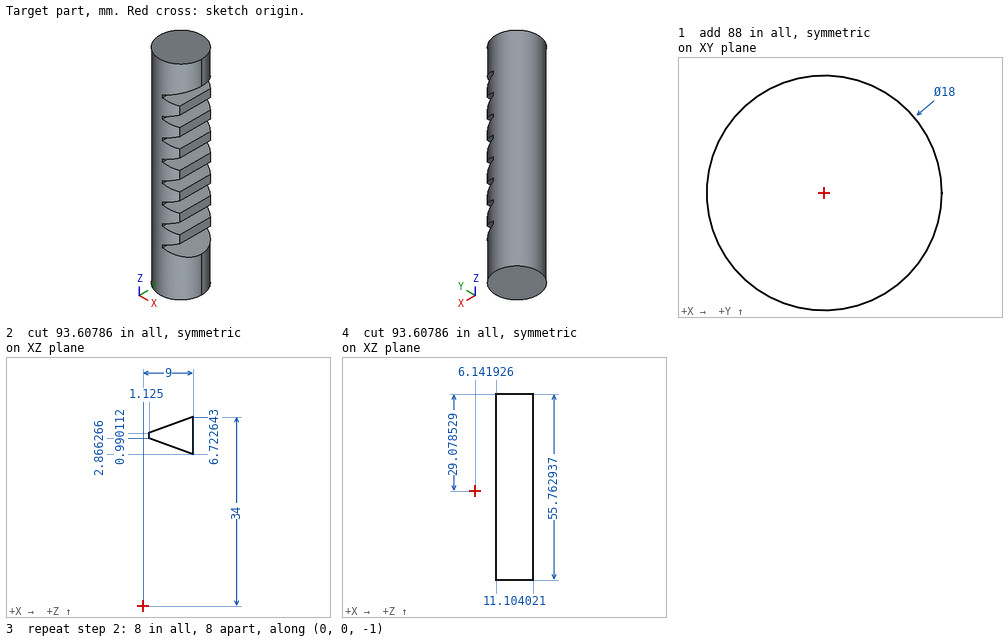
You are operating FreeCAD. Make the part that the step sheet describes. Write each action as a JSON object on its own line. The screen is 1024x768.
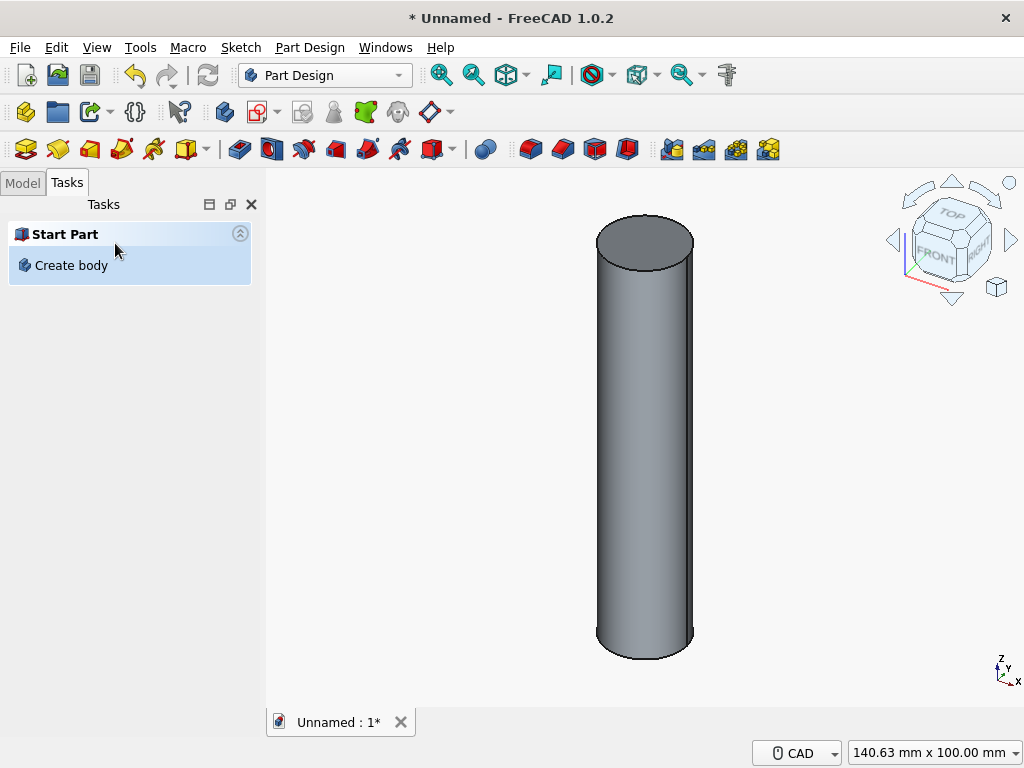
{"action": "left_click", "coordinate": [258, 112]}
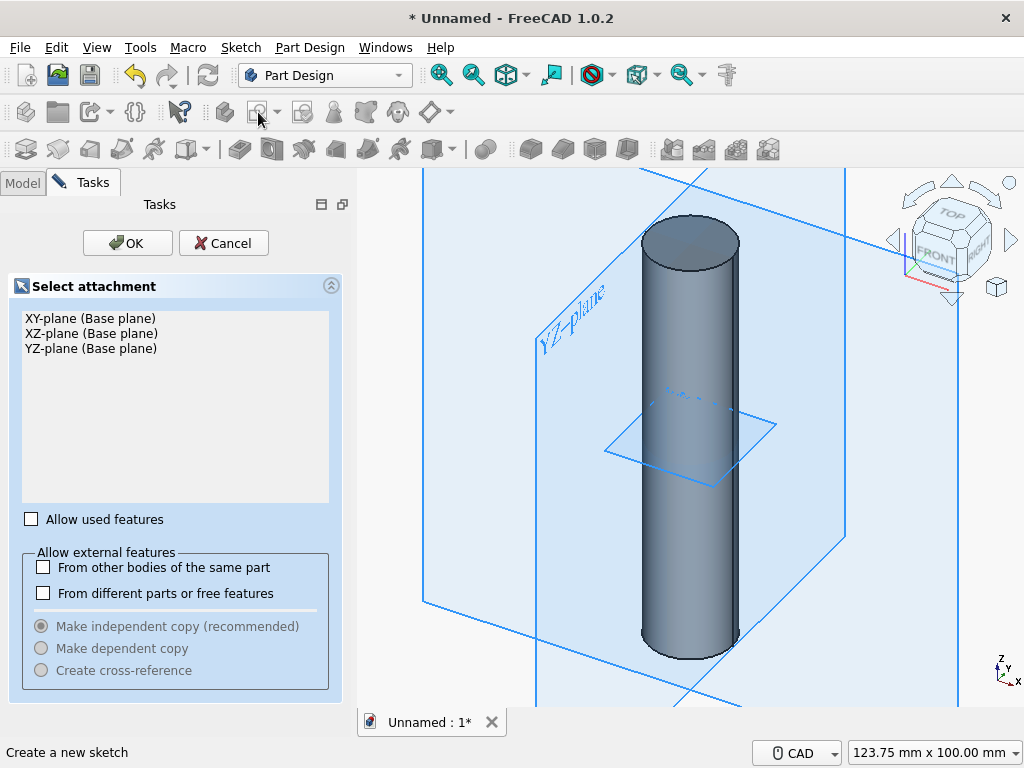
{"action": "left_click", "coordinate": [82, 334]}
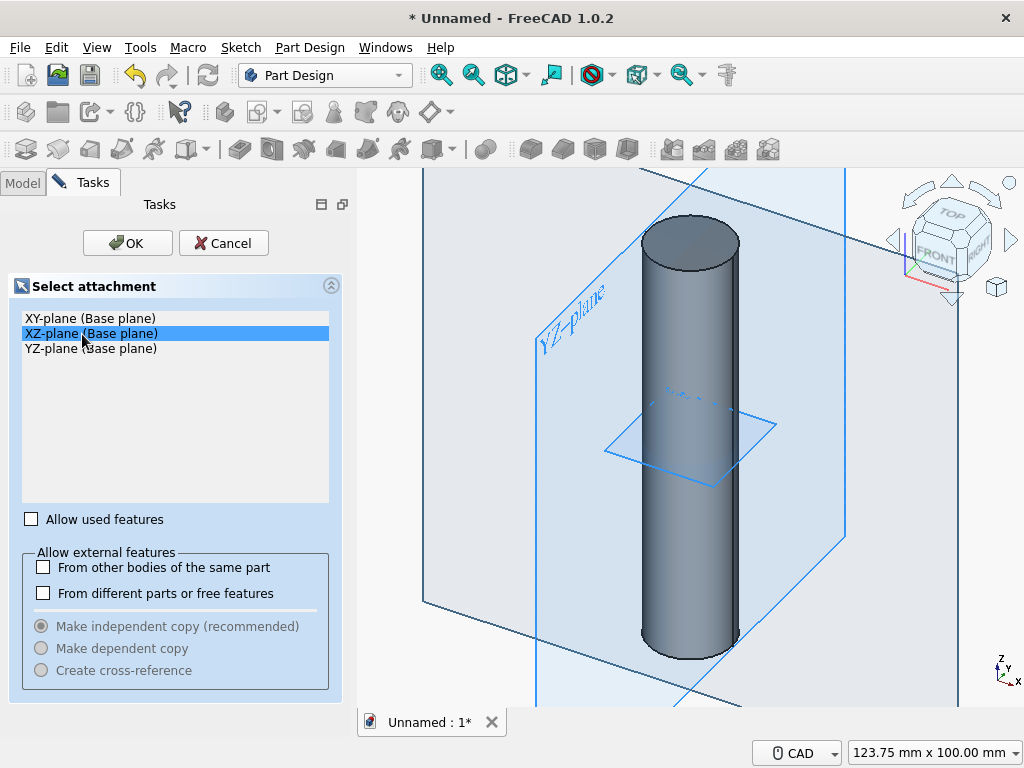
{"action": "left_click", "coordinate": [128, 243]}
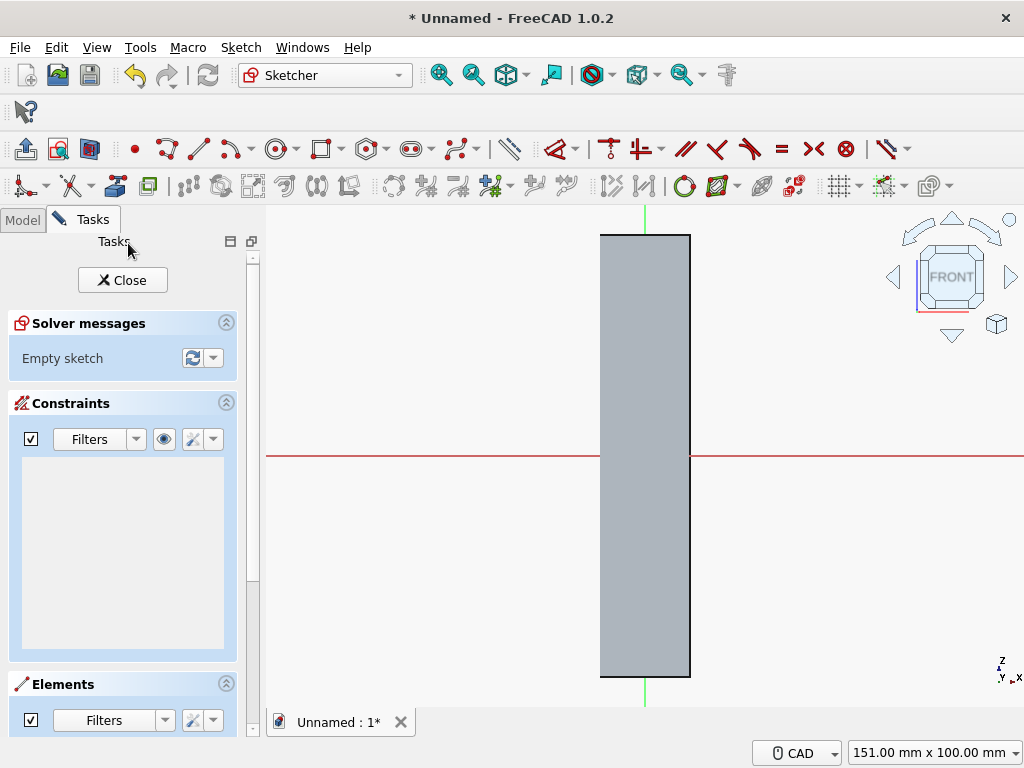
{"action": "left_click", "coordinate": [90, 150]}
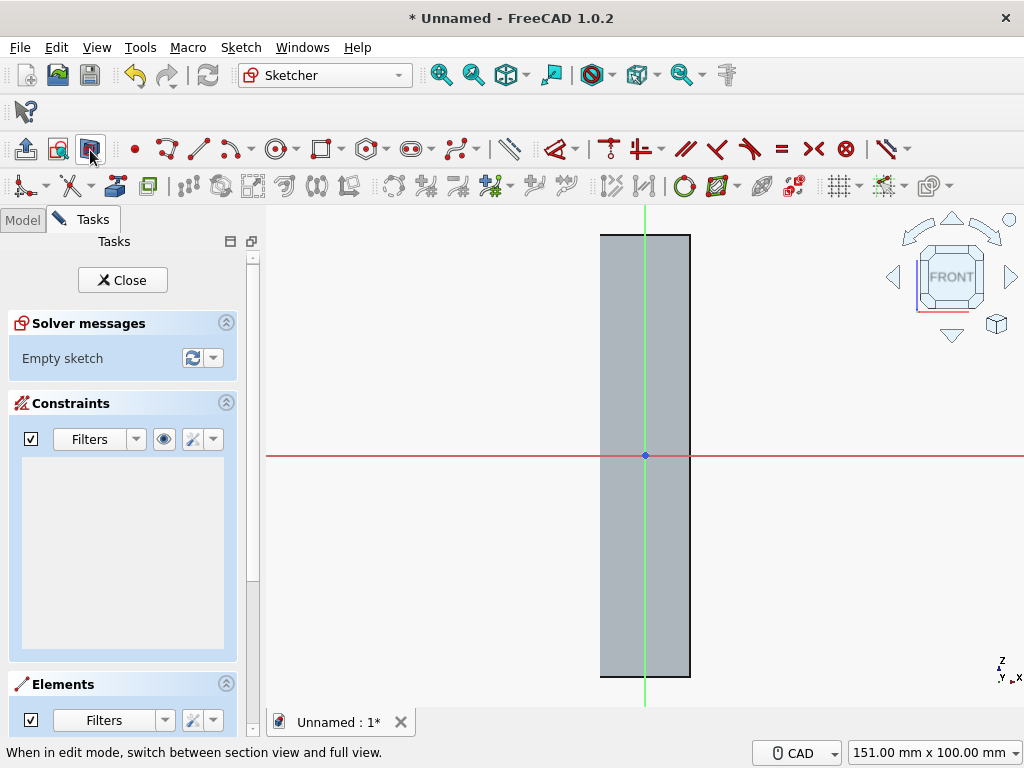
{"action": "scroll", "coordinate": [682, 283], "scroll_direction": "up", "scroll_amount": 11}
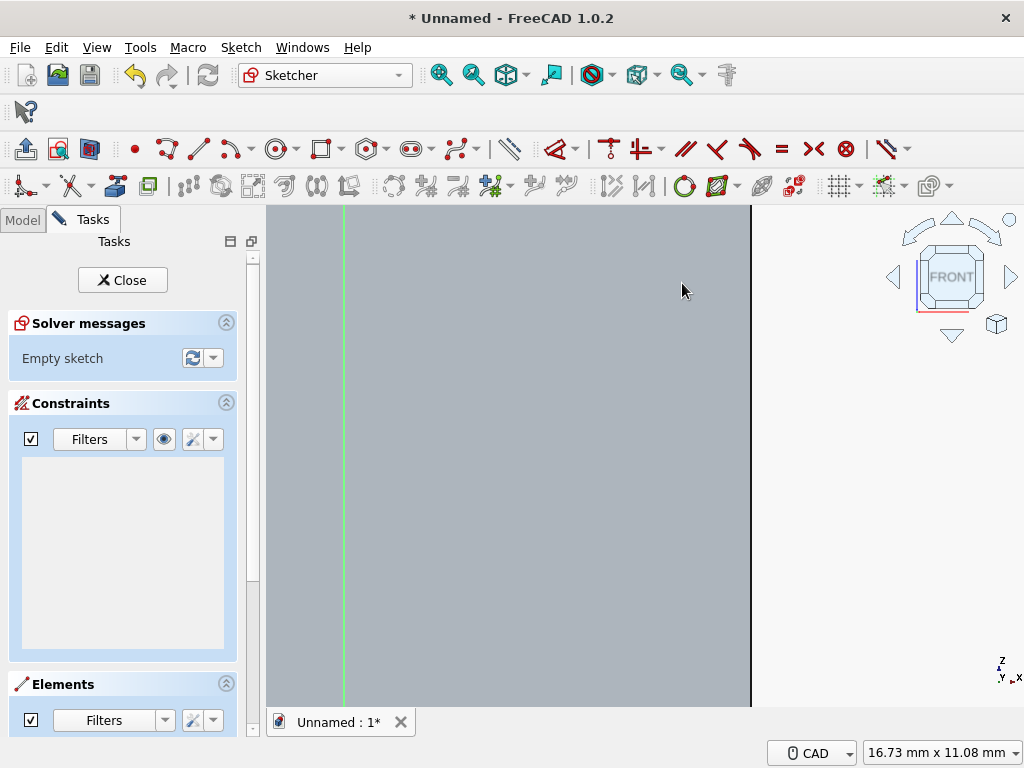
{"action": "key", "text": "g m"}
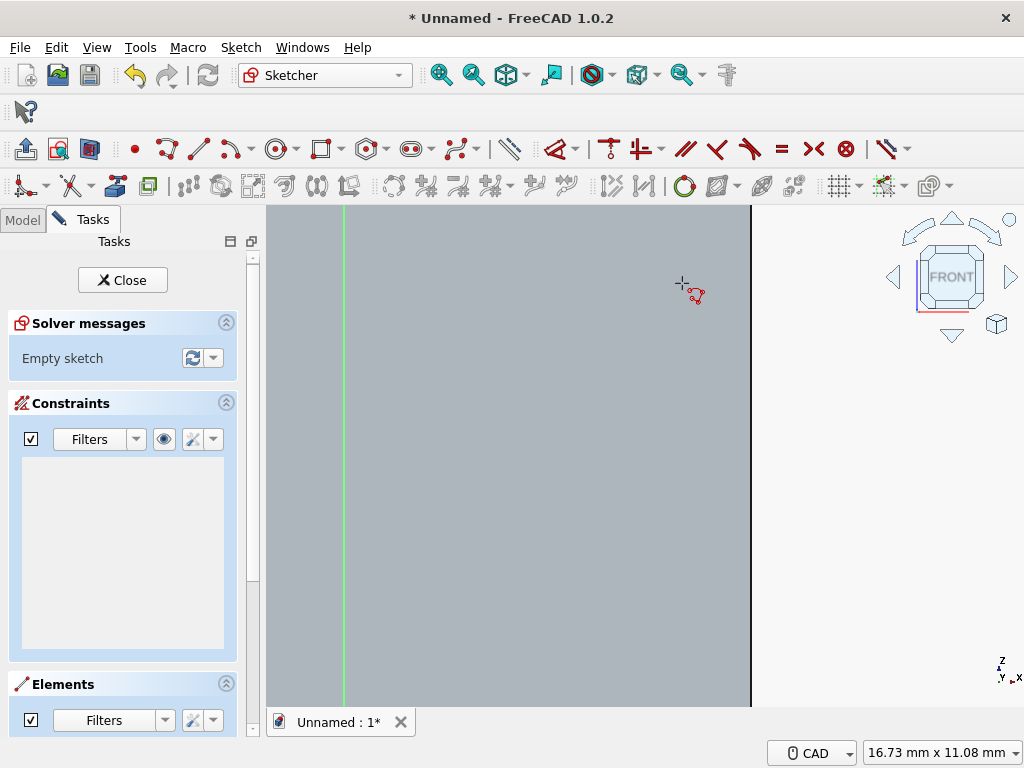
{"action": "left_click", "coordinate": [751, 607]}
{"action": "left_click", "coordinate": [395, 477]}
{"action": "left_click", "coordinate": [395, 433]}
{"action": "left_click", "coordinate": [751, 303]}
{"action": "left_click", "coordinate": [751, 608]}
{"action": "key", "text": "Escape"}
{"action": "key", "text": "Escape"}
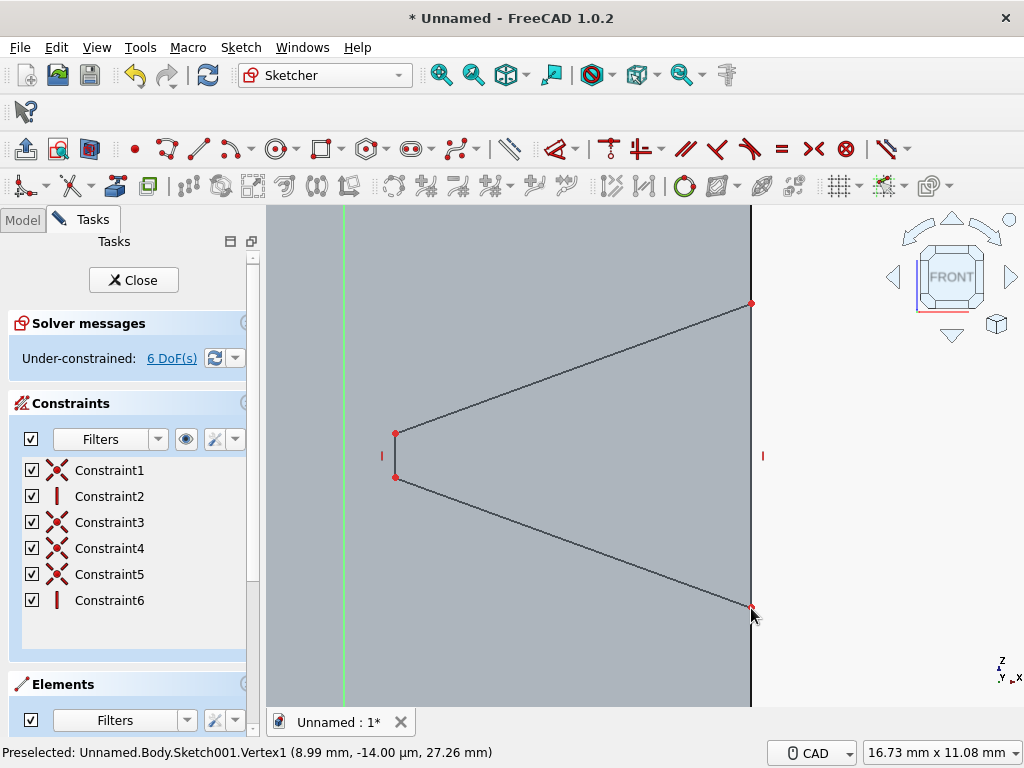
{"action": "left_click", "coordinate": [751, 608]}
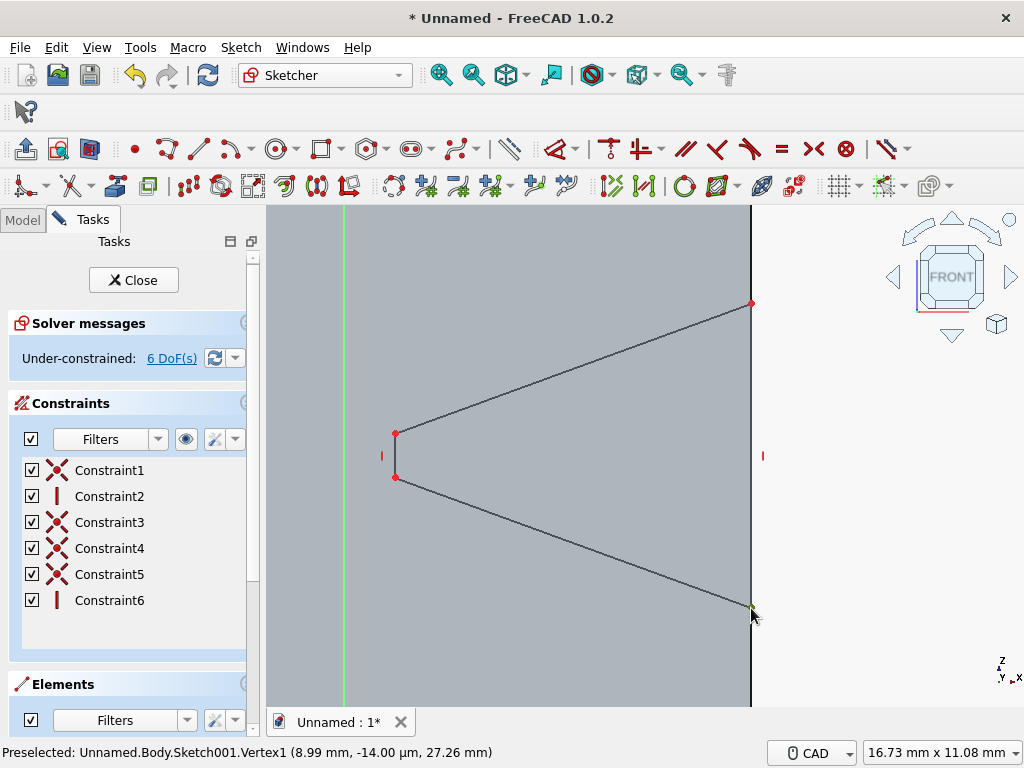
{"action": "left_click", "coordinate": [578, 150]}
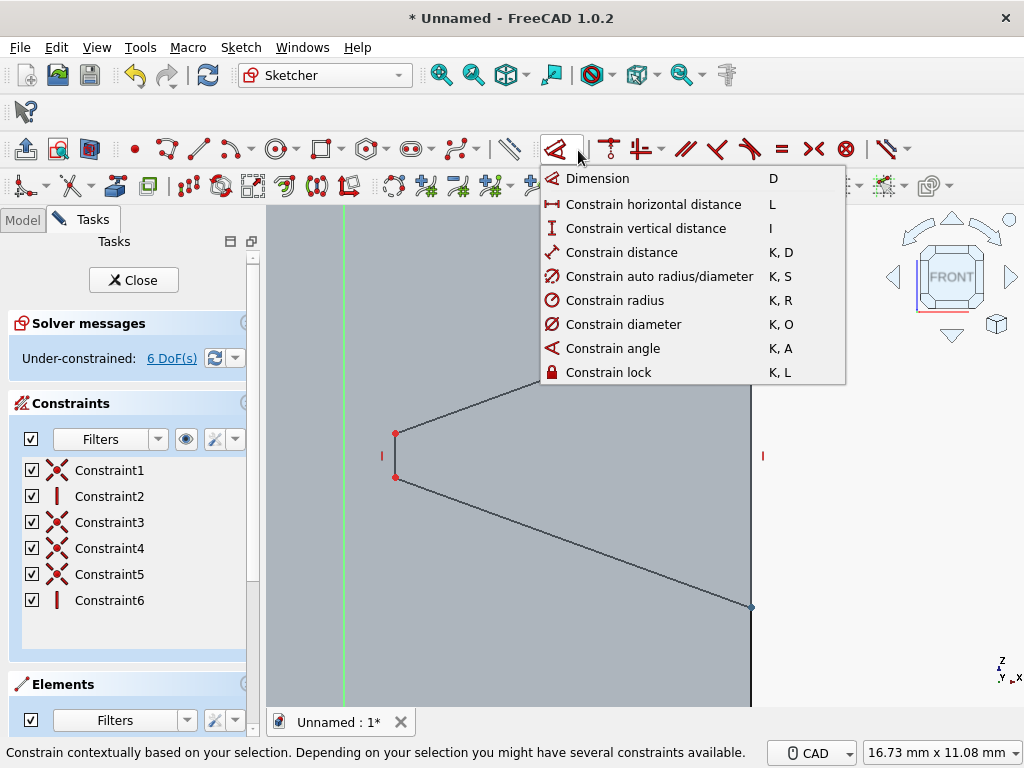
{"action": "left_click", "coordinate": [693, 204]}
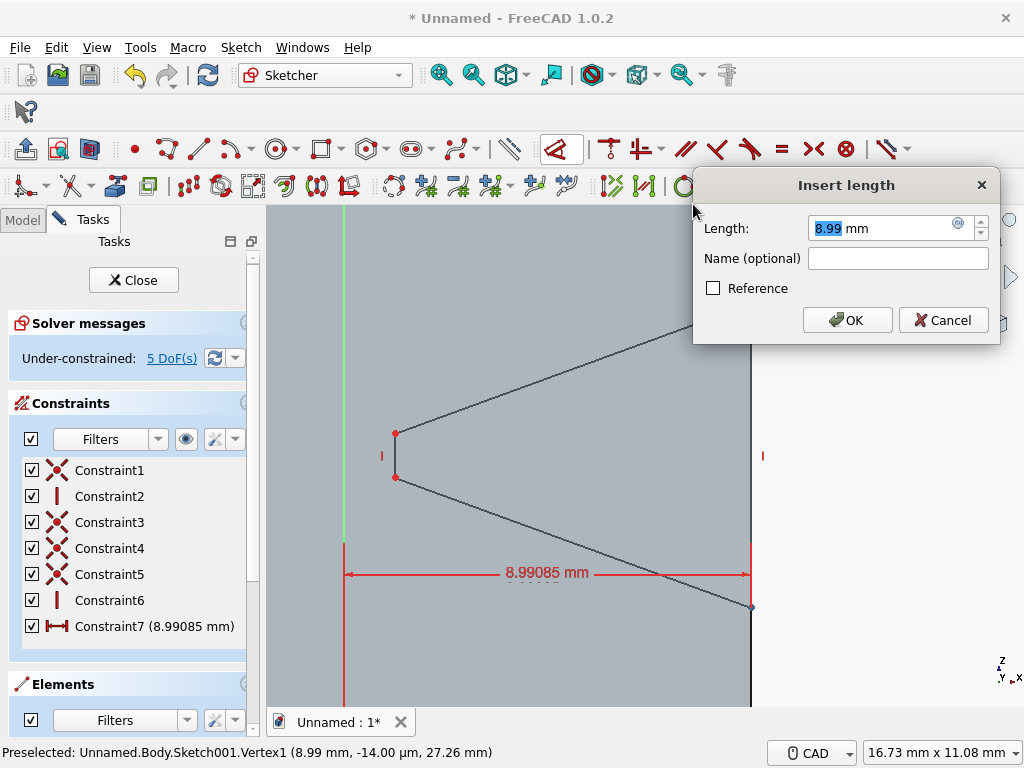
{"action": "type", "text": "9"}
{"action": "key", "text": "Return"}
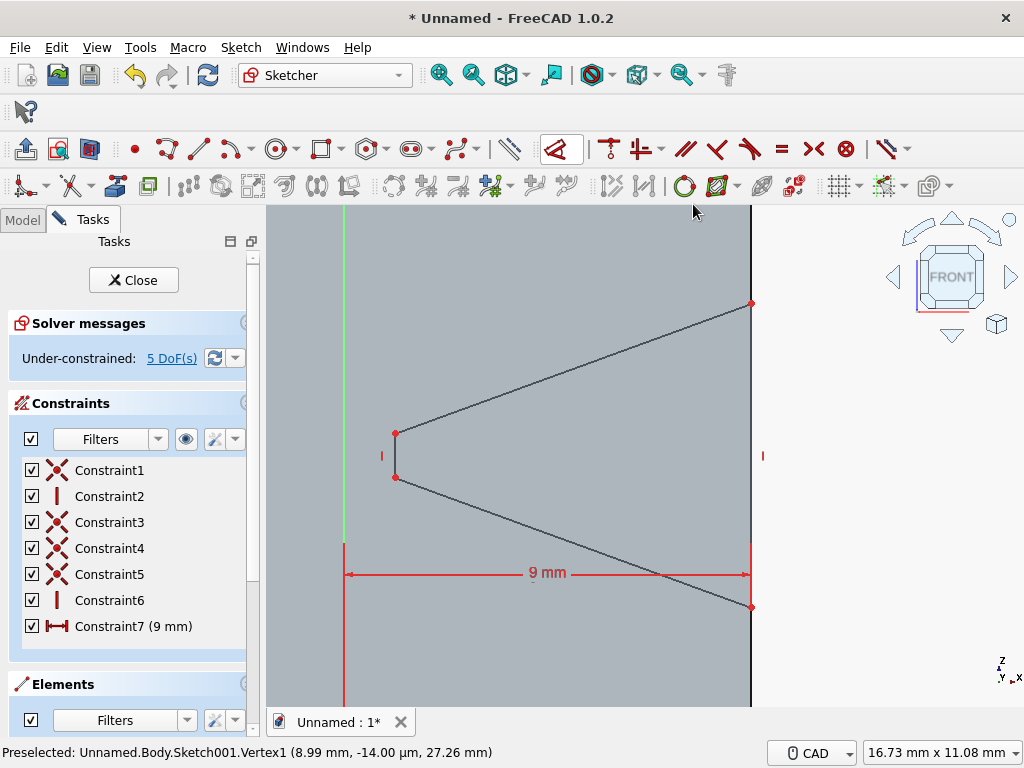
{"action": "left_click", "coordinate": [751, 304]}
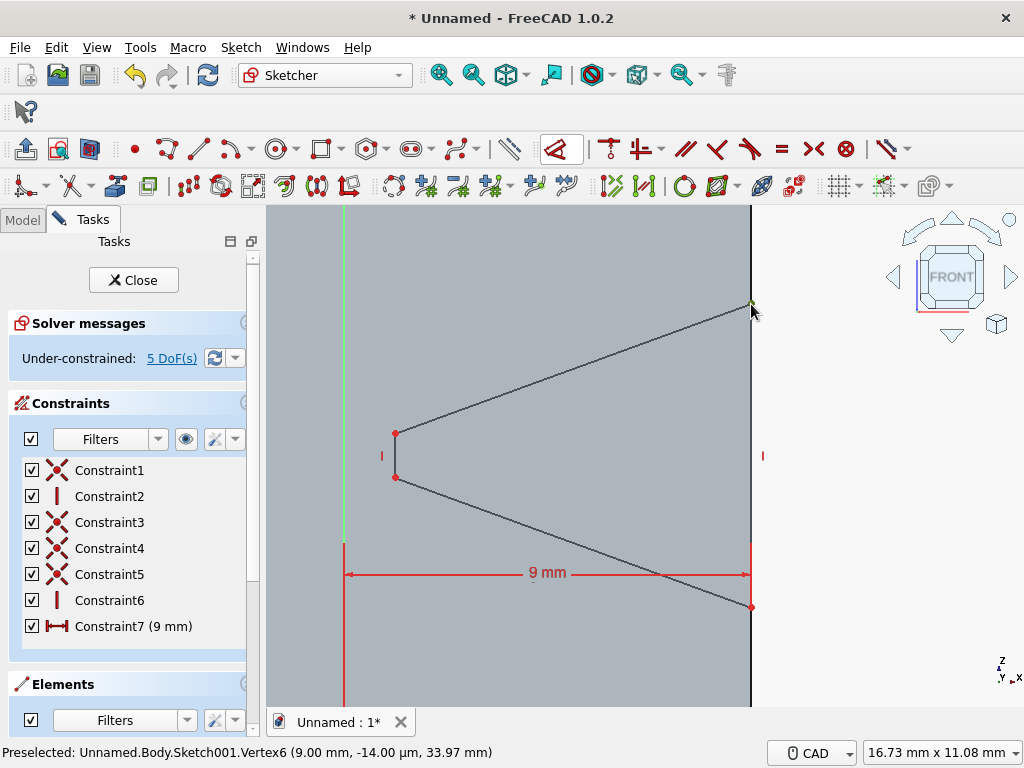
{"action": "key", "text": "i"}